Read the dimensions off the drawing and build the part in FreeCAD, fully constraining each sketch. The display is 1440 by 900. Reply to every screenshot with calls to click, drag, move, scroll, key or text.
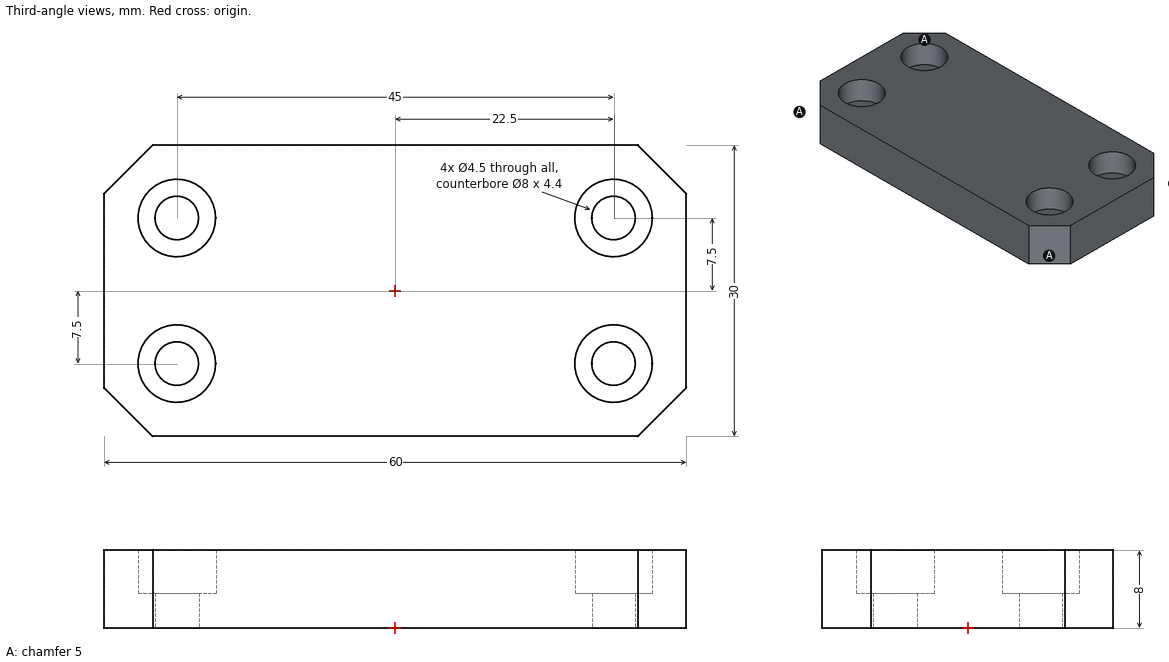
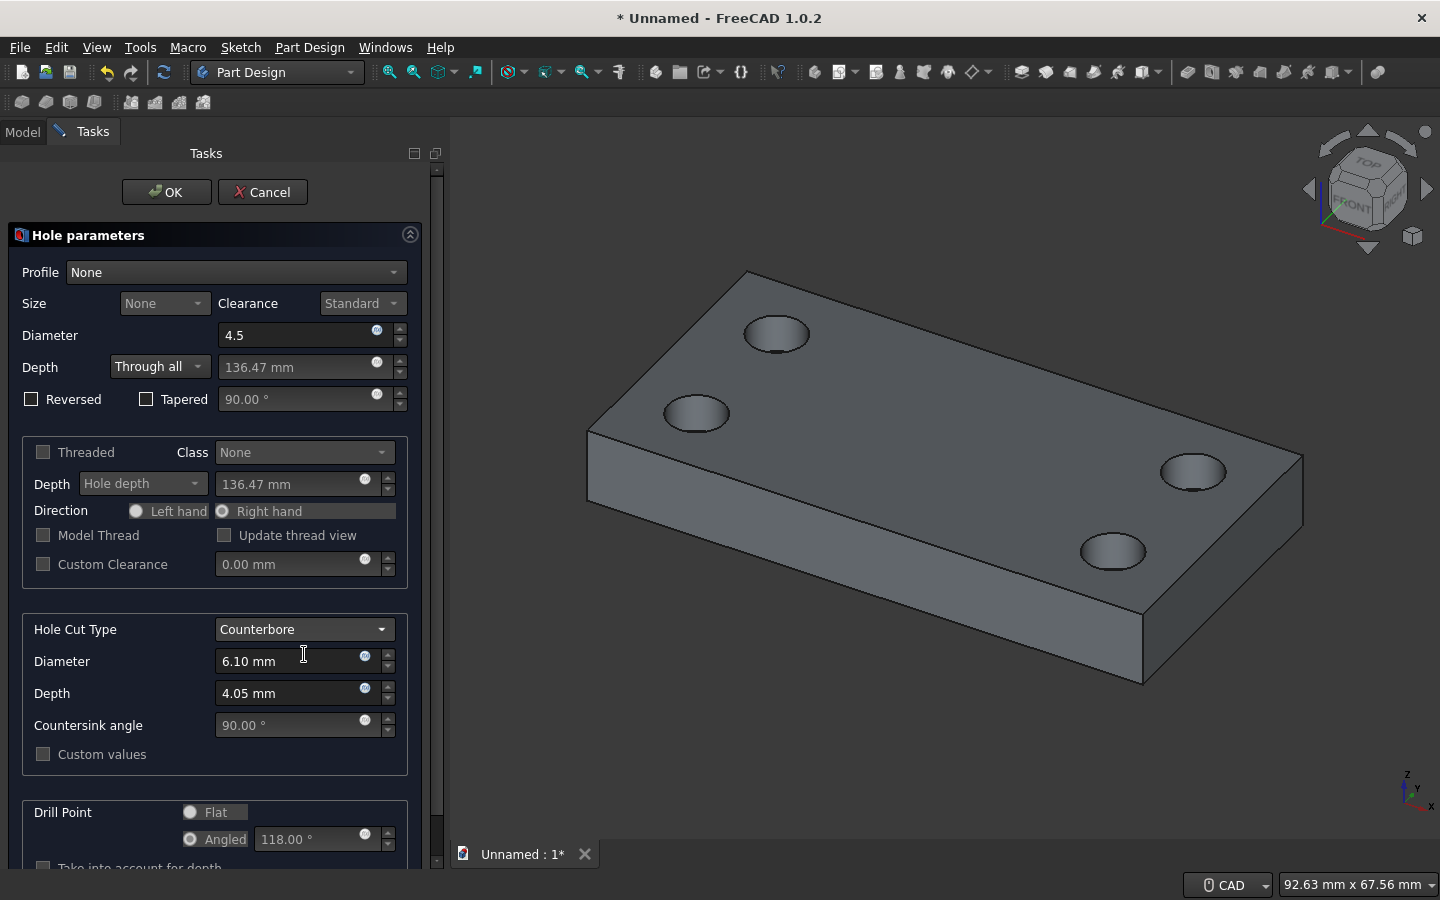
triple_click(298, 661)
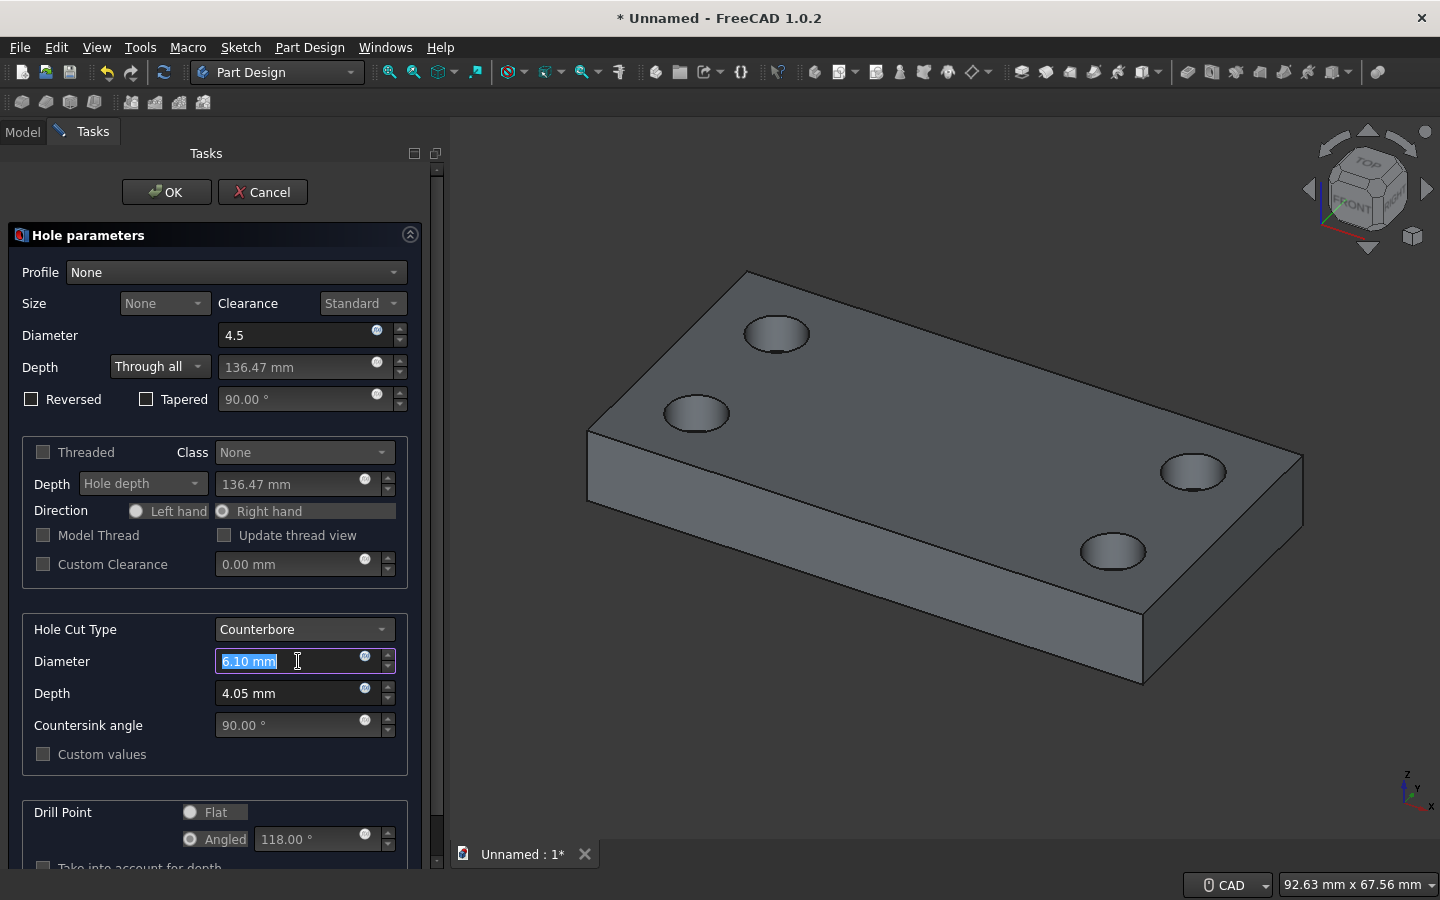
text(8)
key(Tab)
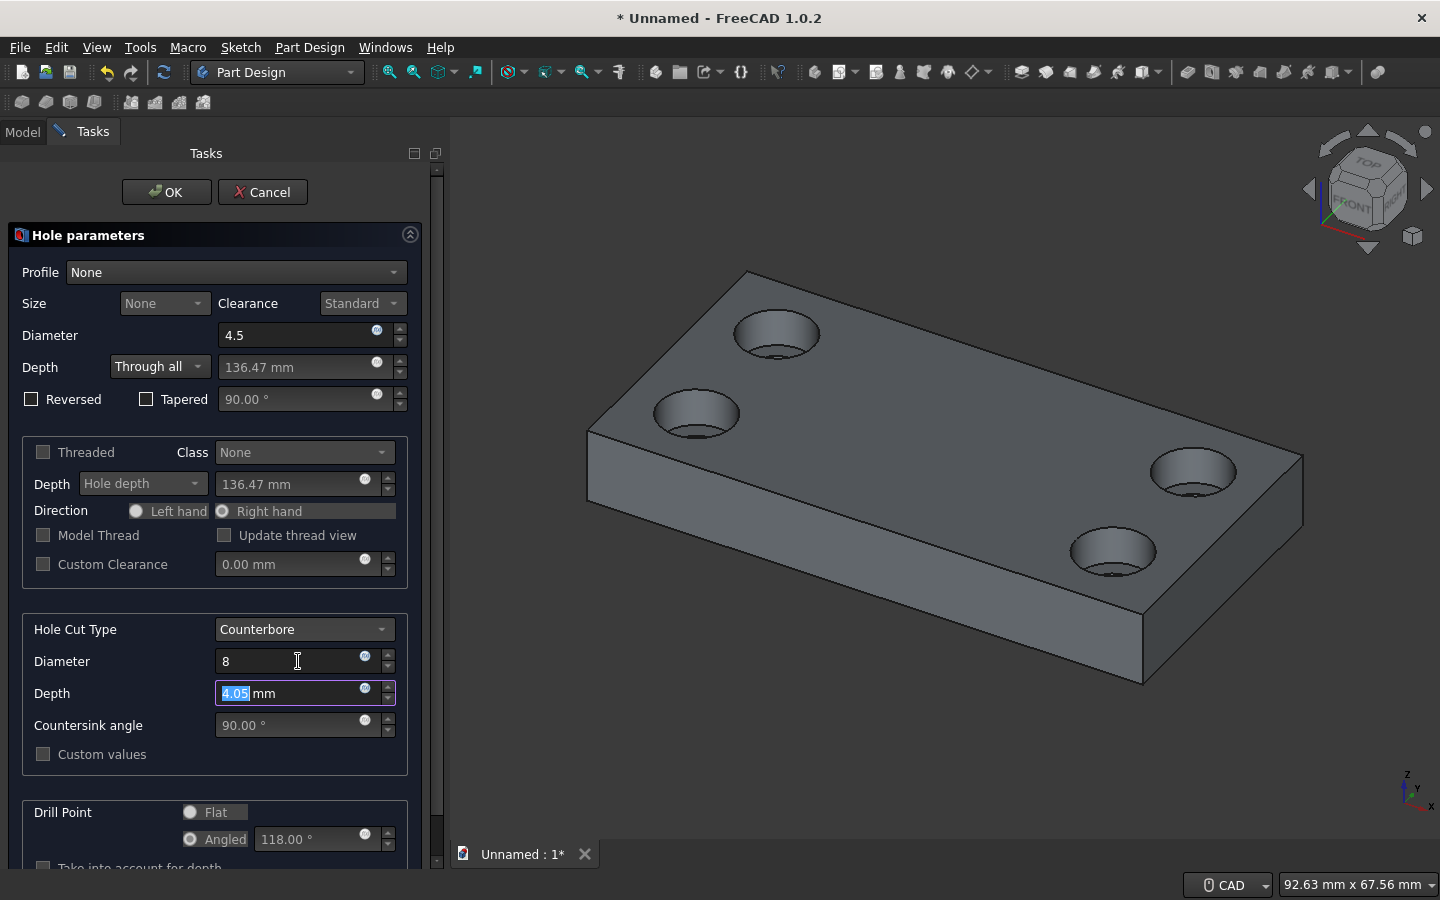
text(4.4)
key(Tab)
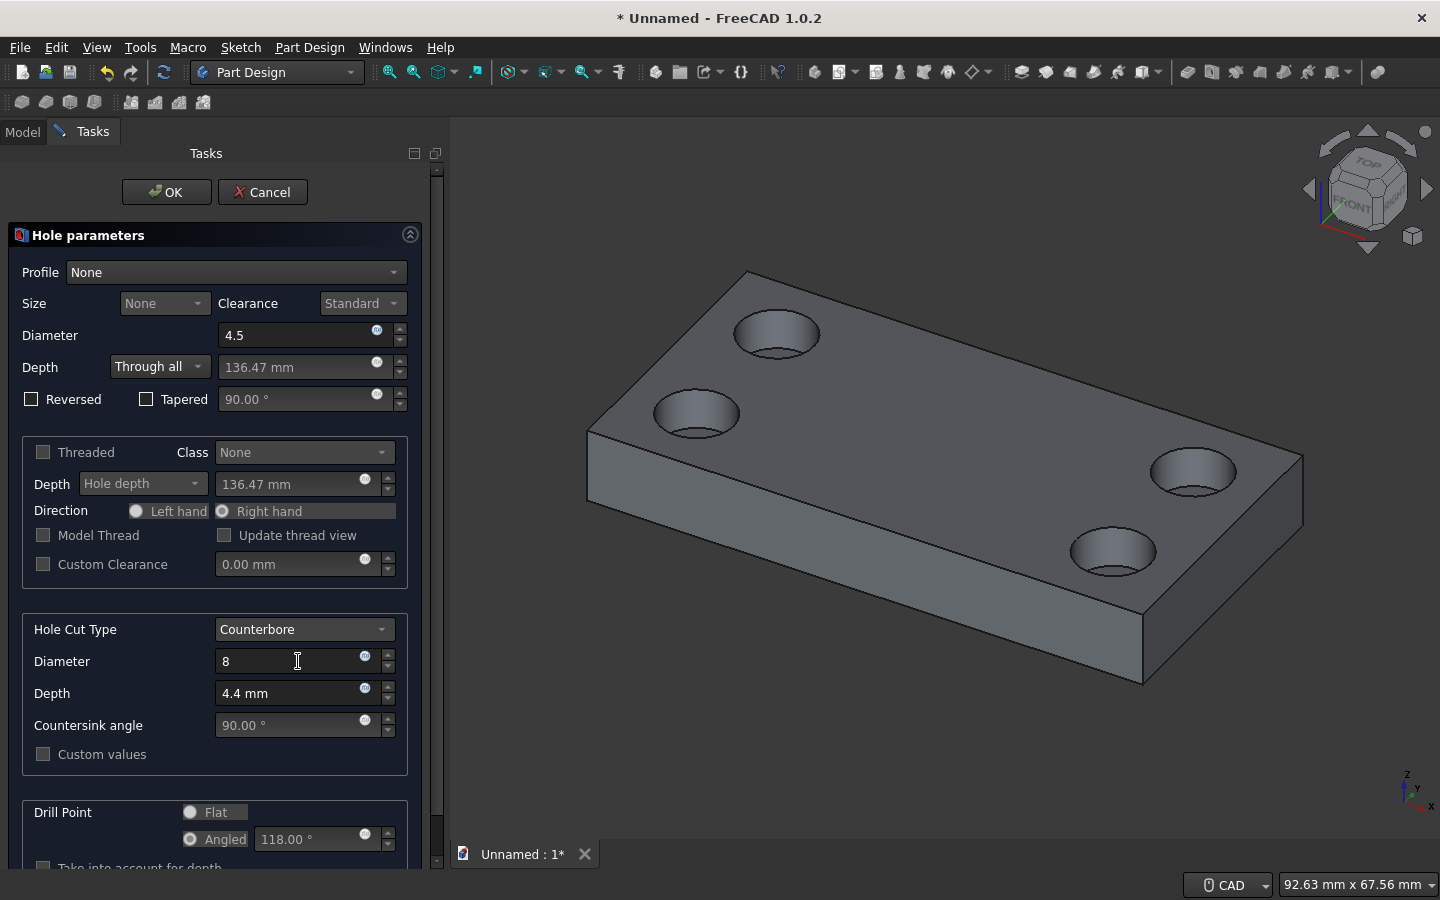
click(167, 192)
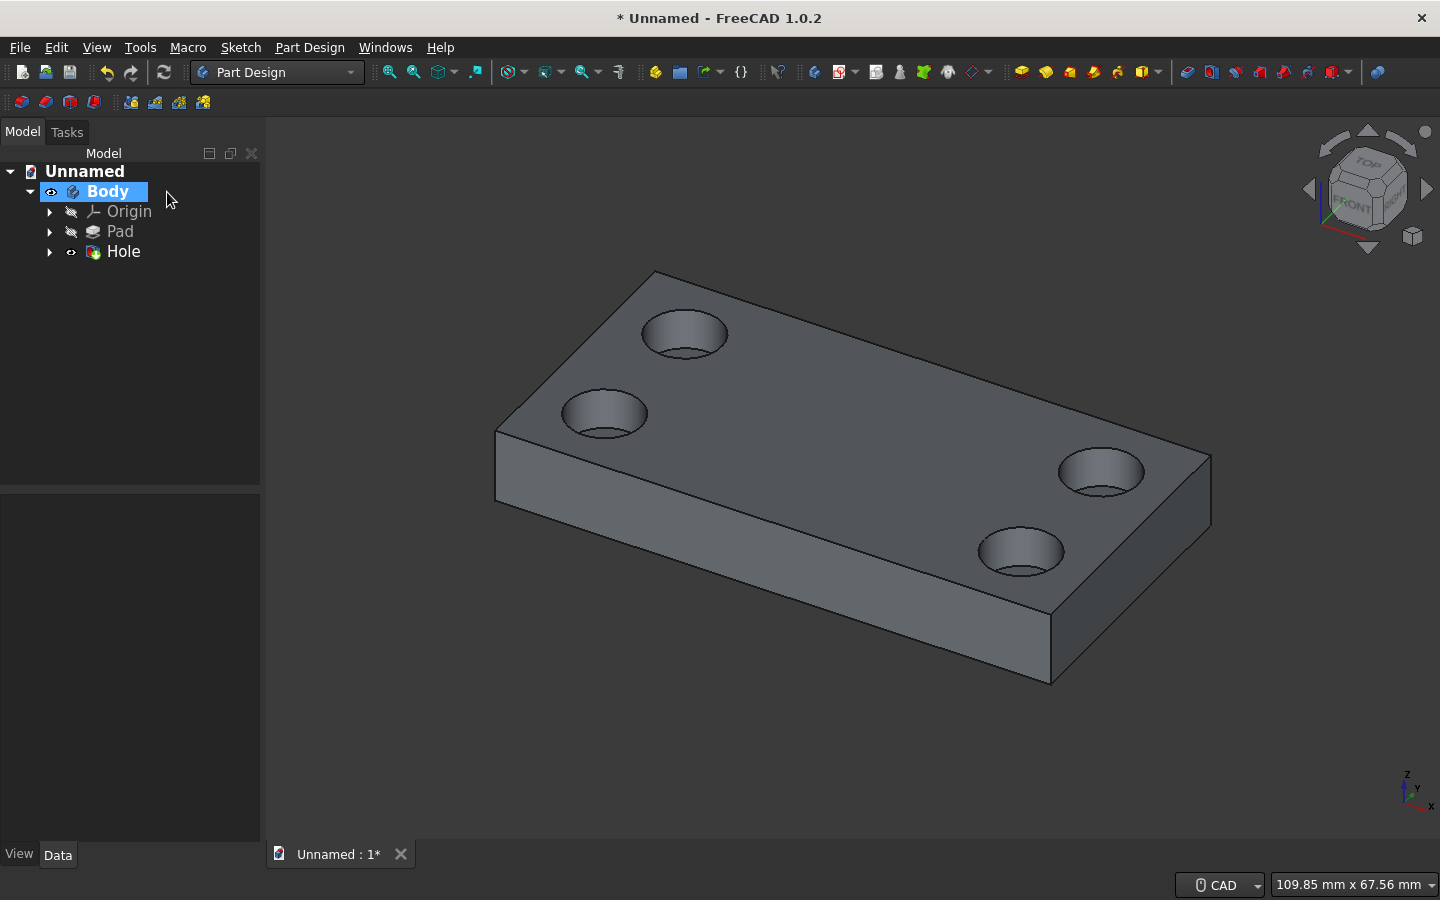
click(1051, 649)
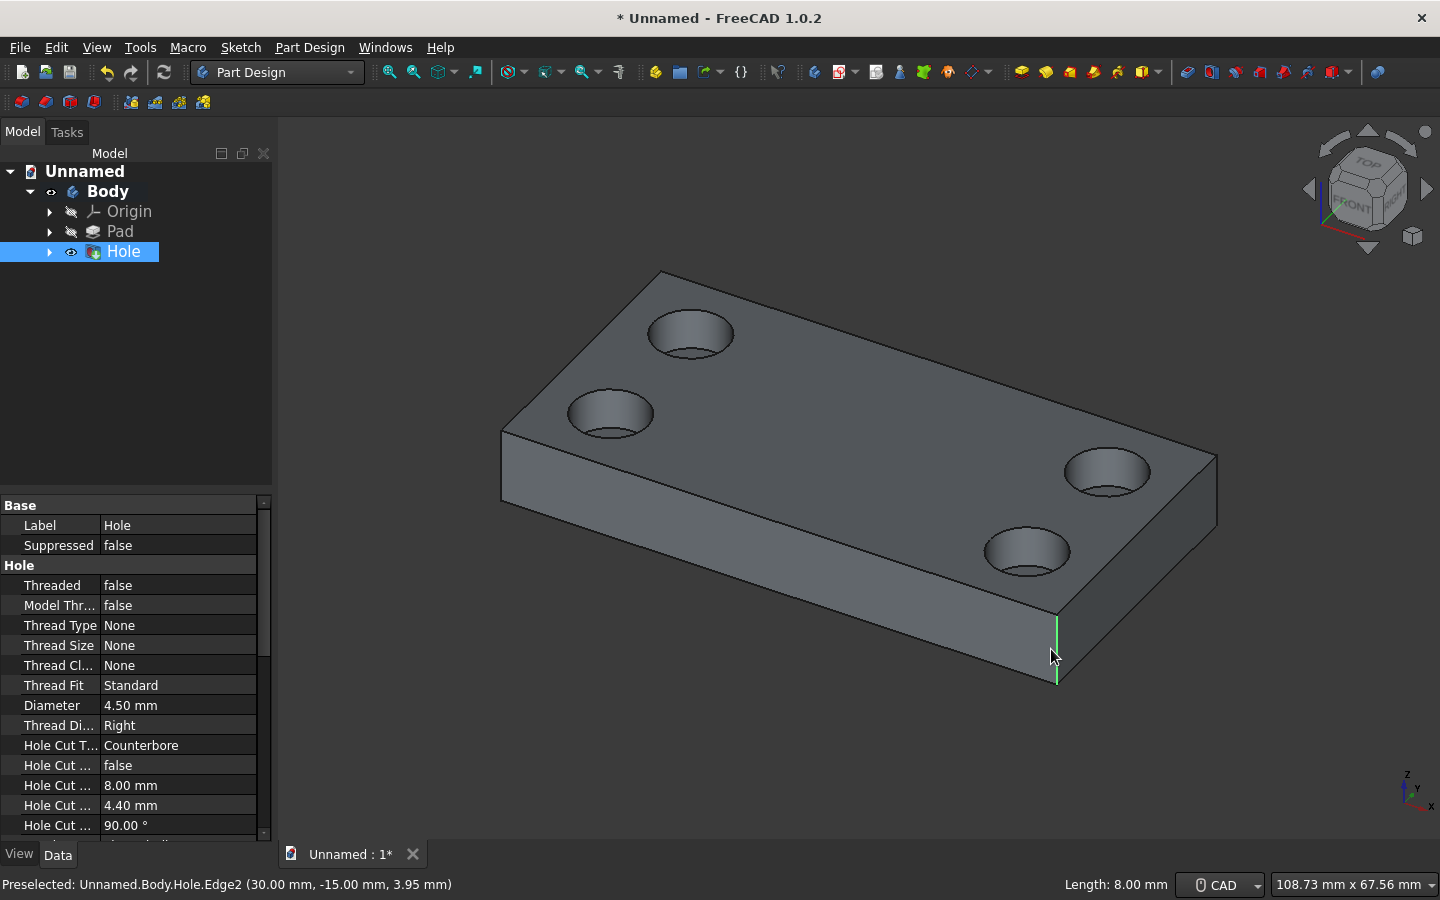
key(0)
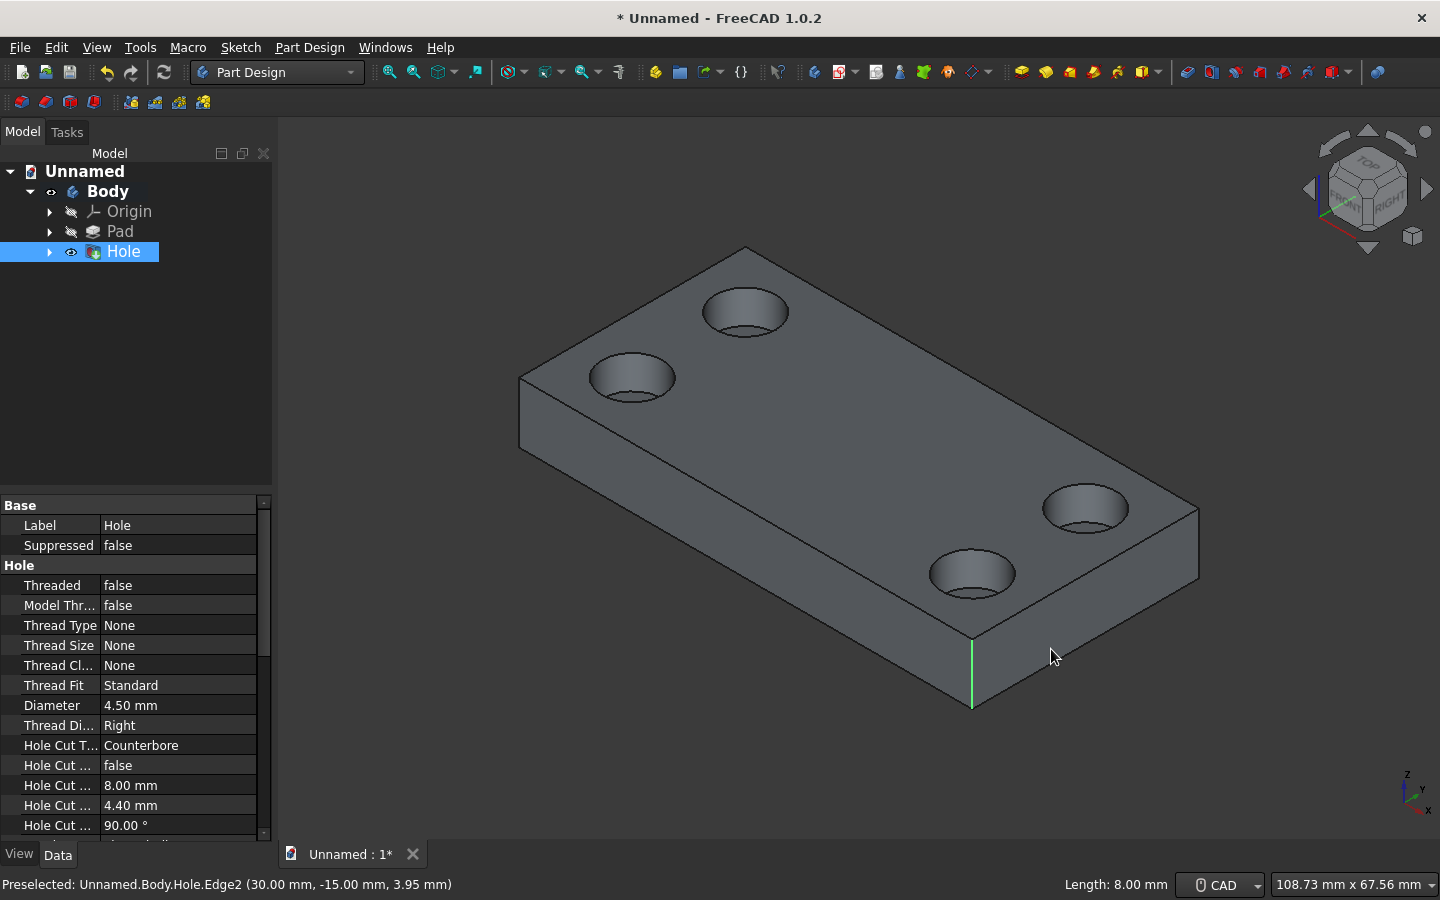
key(2)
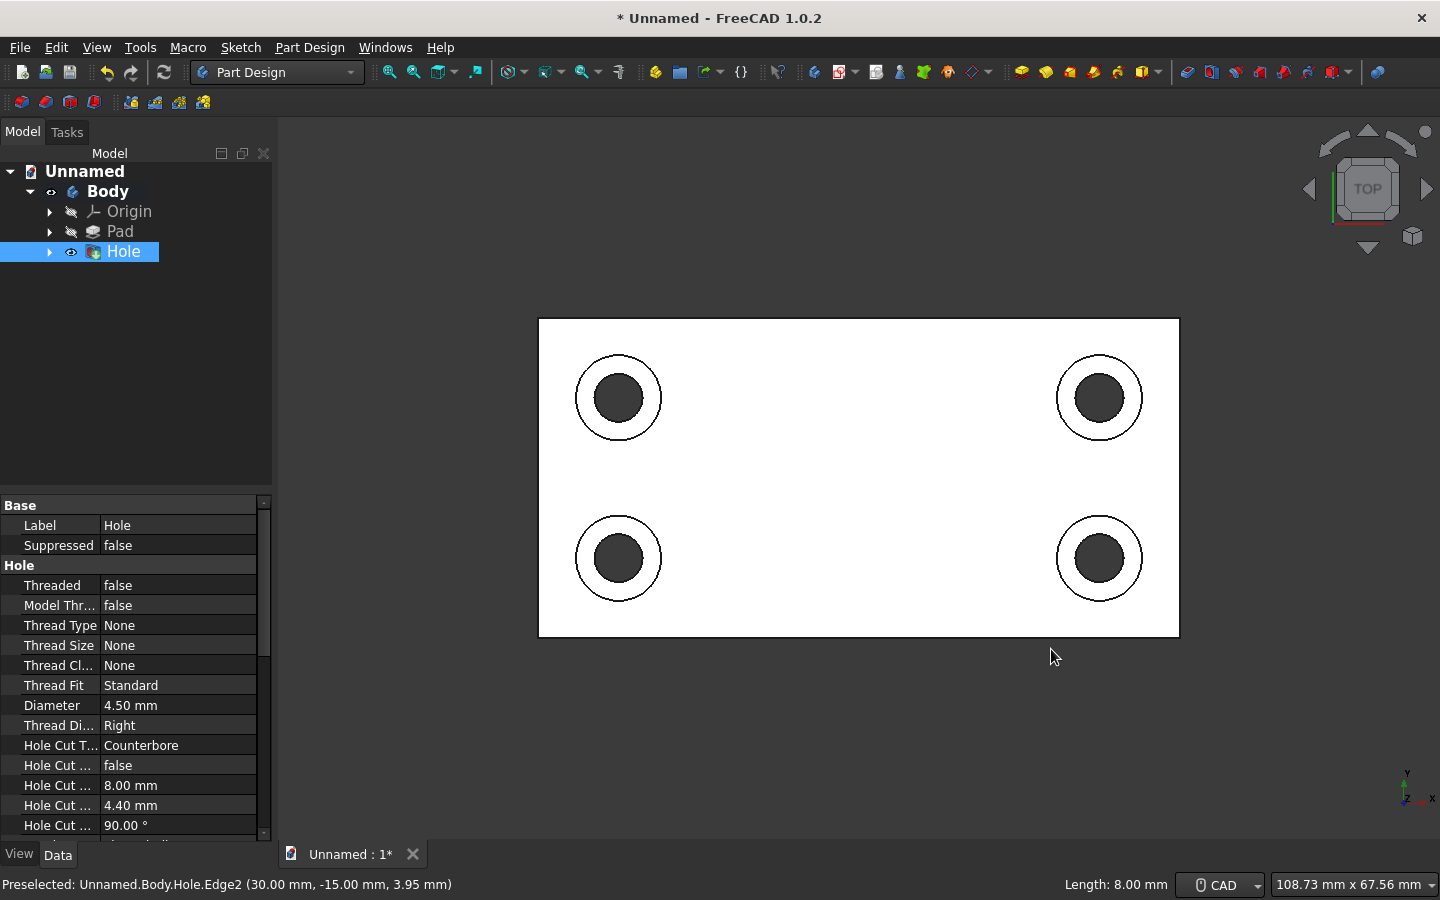
key(1)